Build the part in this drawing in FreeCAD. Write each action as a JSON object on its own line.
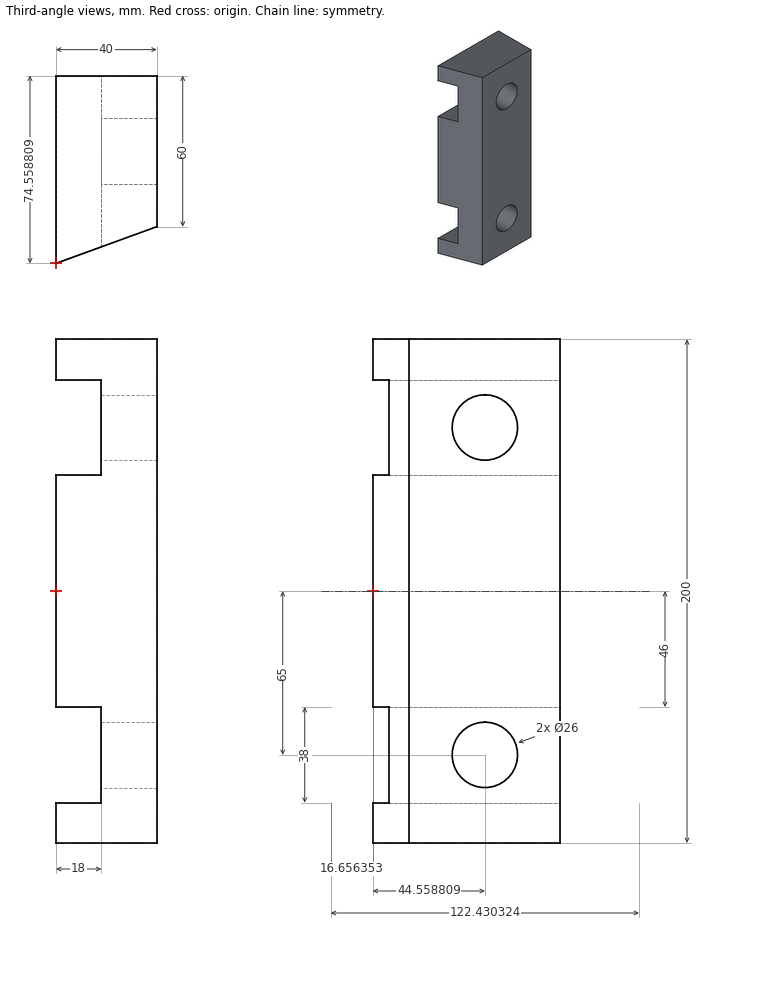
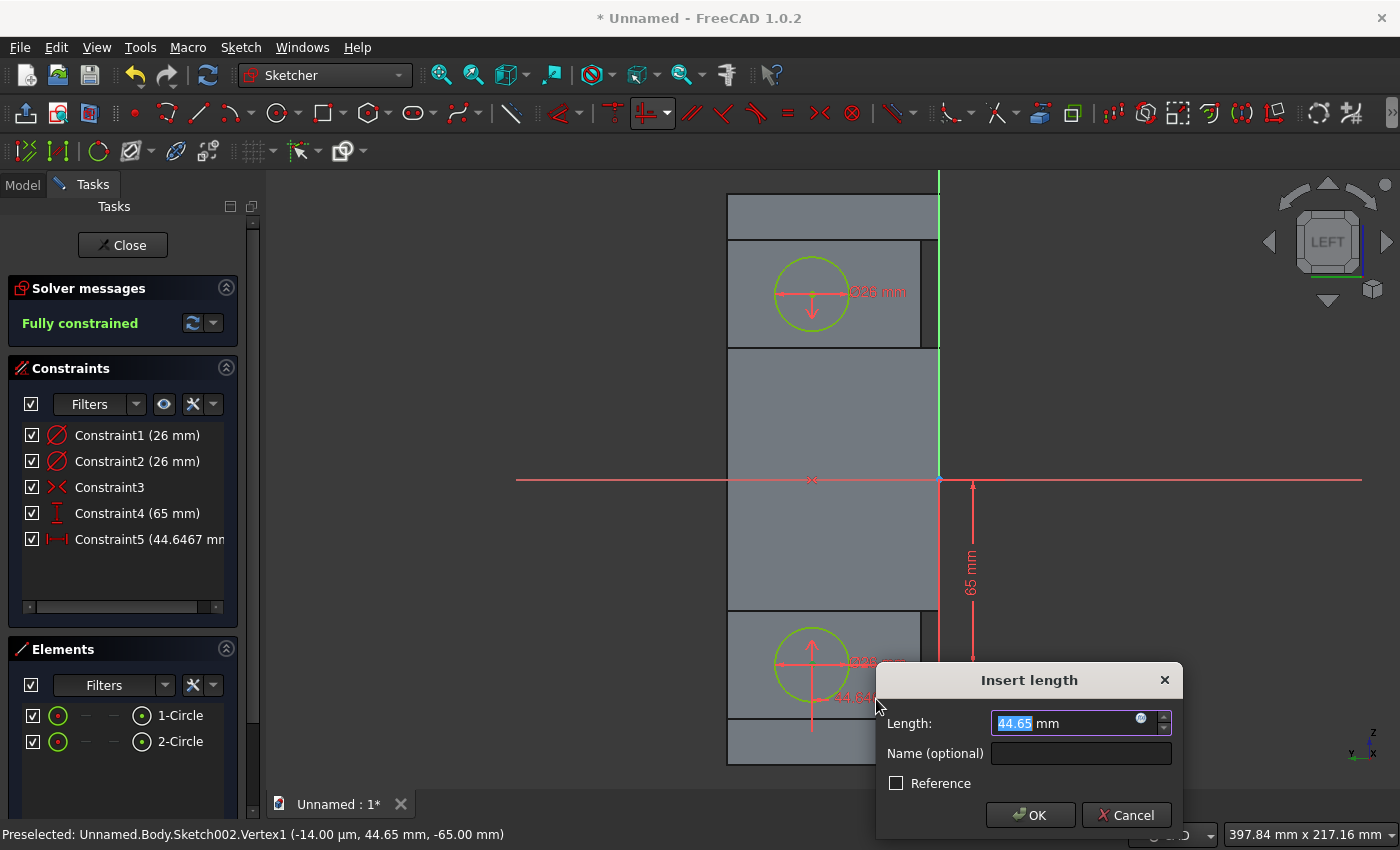
{"action": "type", "text": "44.558809"}
{"action": "key", "text": "Return"}
{"action": "key", "text": "Escape"}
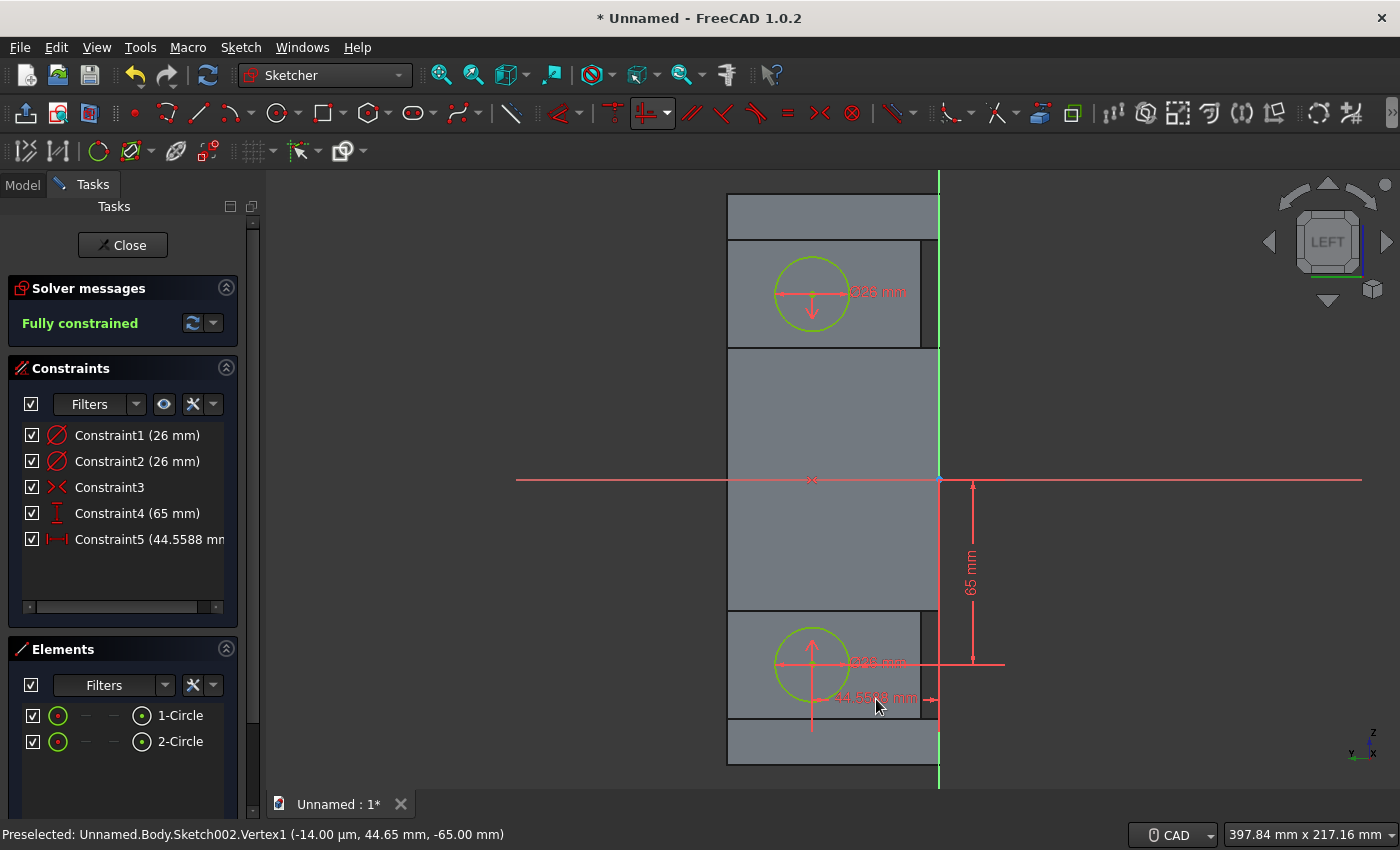
{"action": "left_click", "coordinate": [123, 245]}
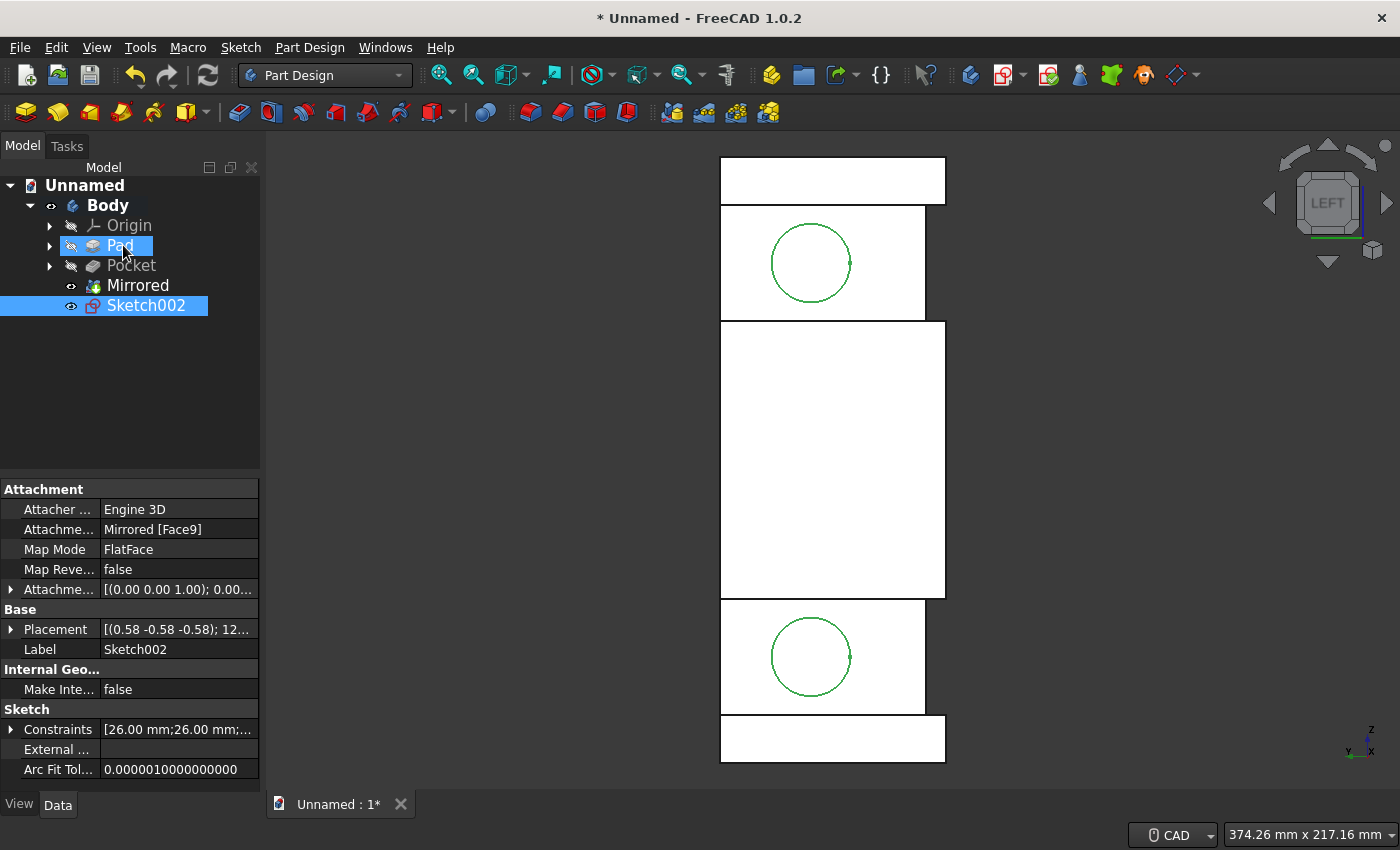
{"action": "left_click", "coordinate": [240, 112]}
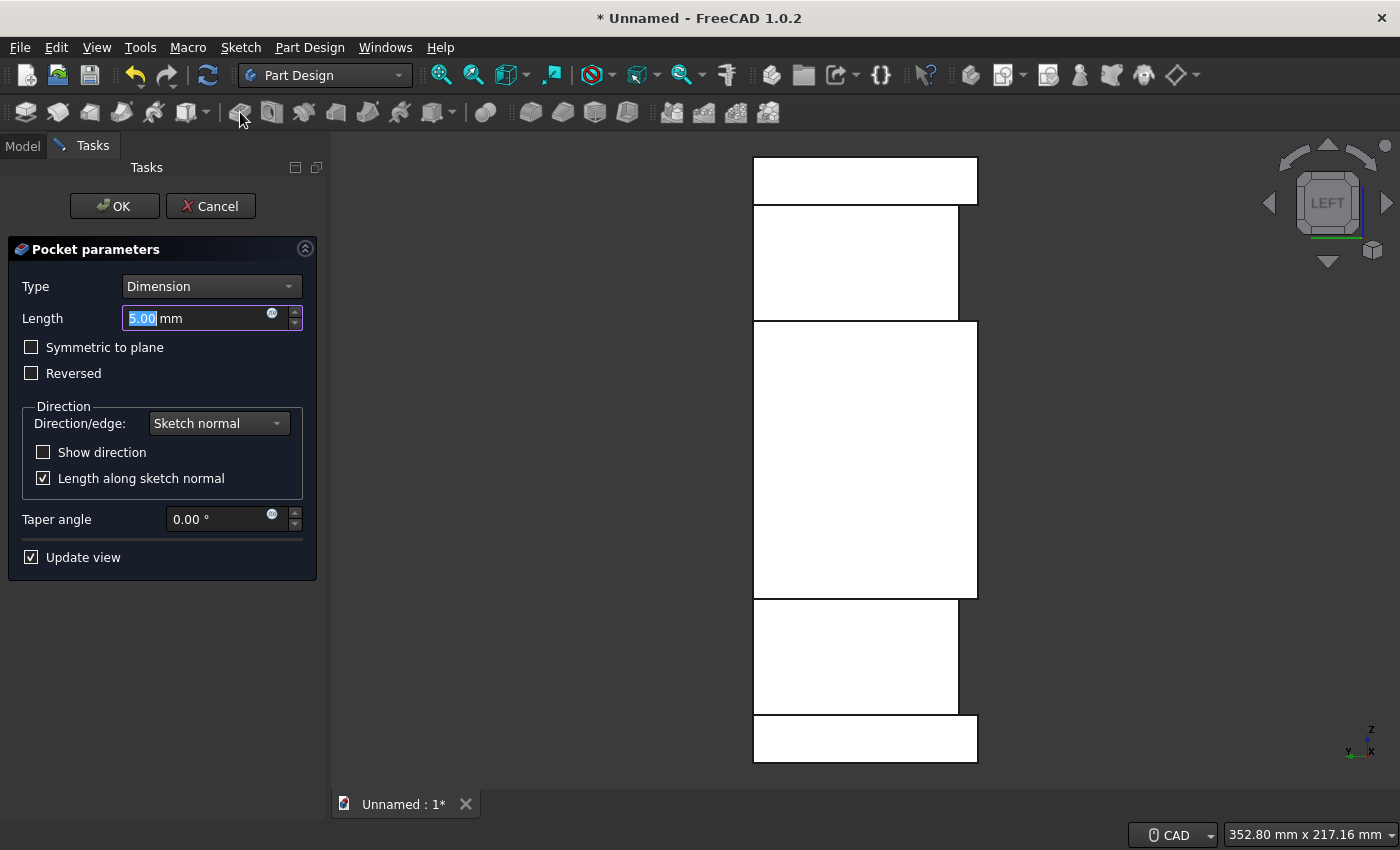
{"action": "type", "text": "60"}
{"action": "key", "text": "Tab"}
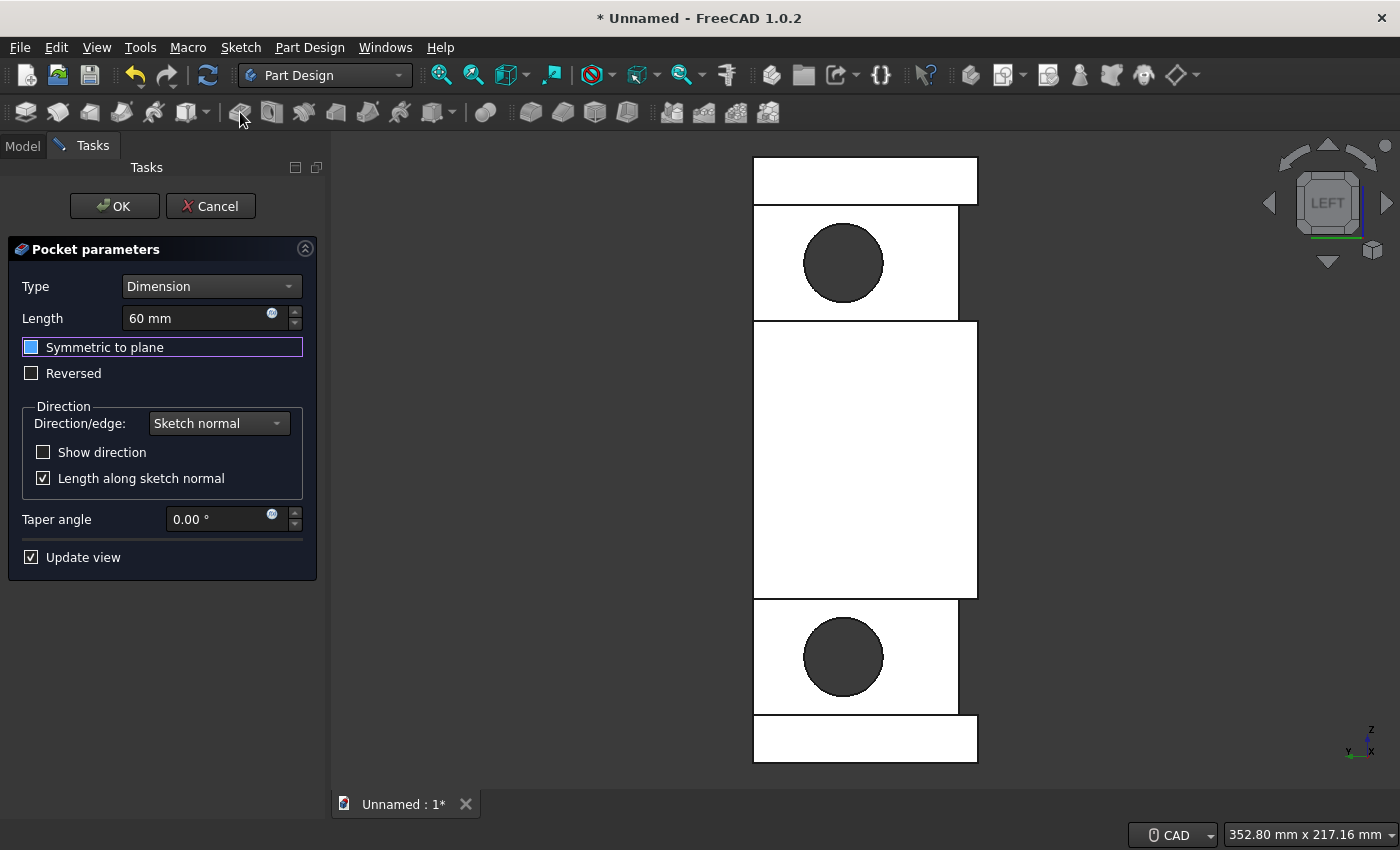
{"action": "left_click", "coordinate": [115, 206]}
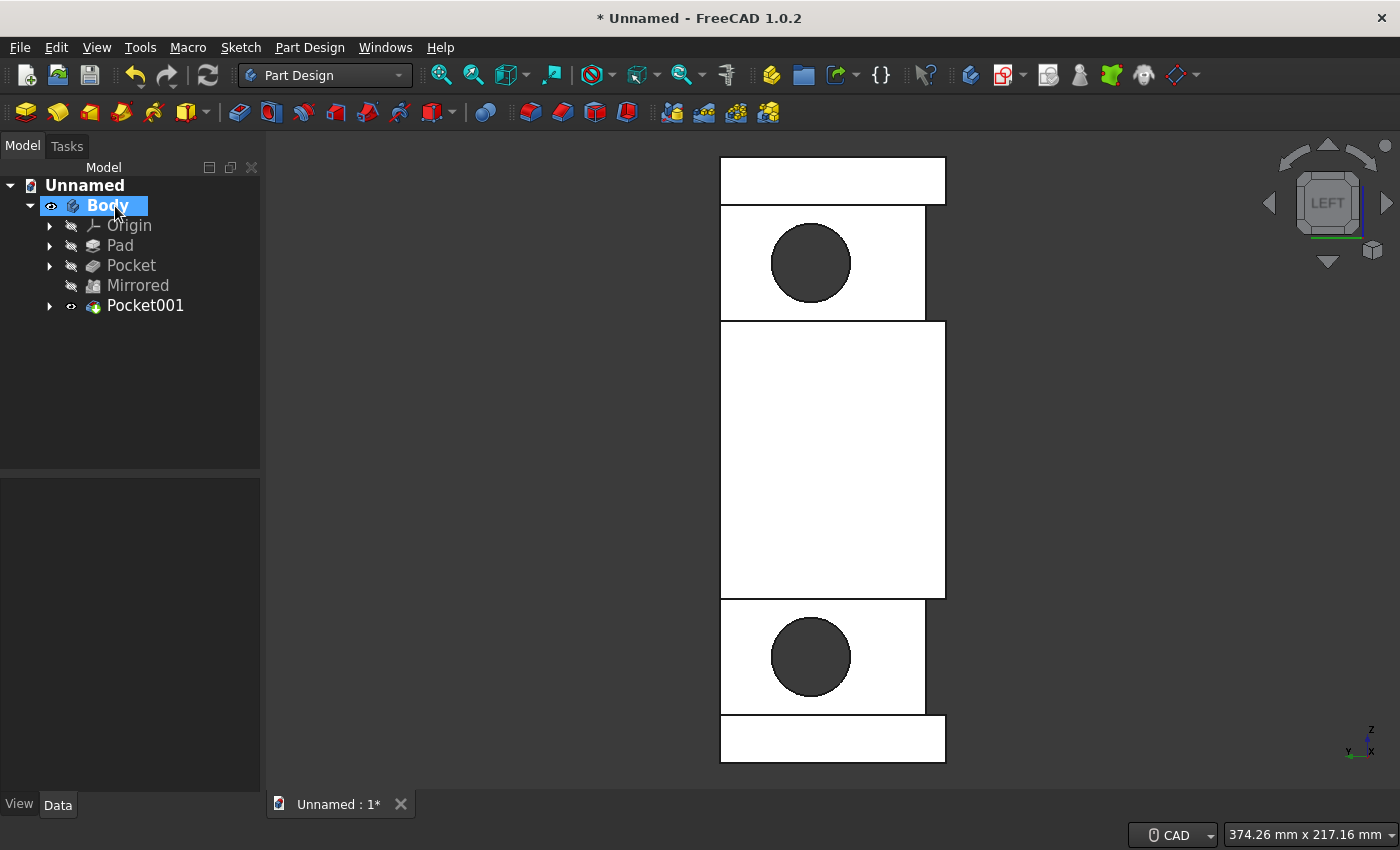
{"action": "key", "text": "0"}